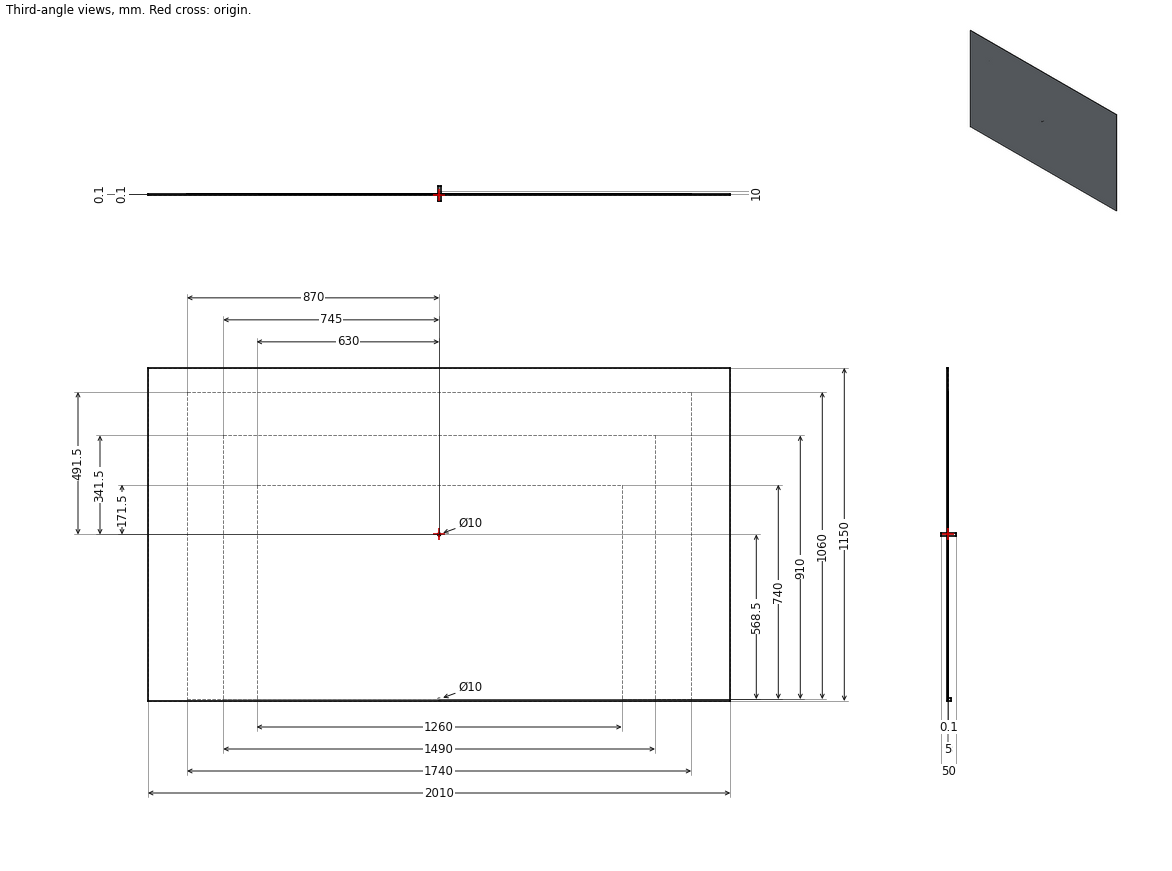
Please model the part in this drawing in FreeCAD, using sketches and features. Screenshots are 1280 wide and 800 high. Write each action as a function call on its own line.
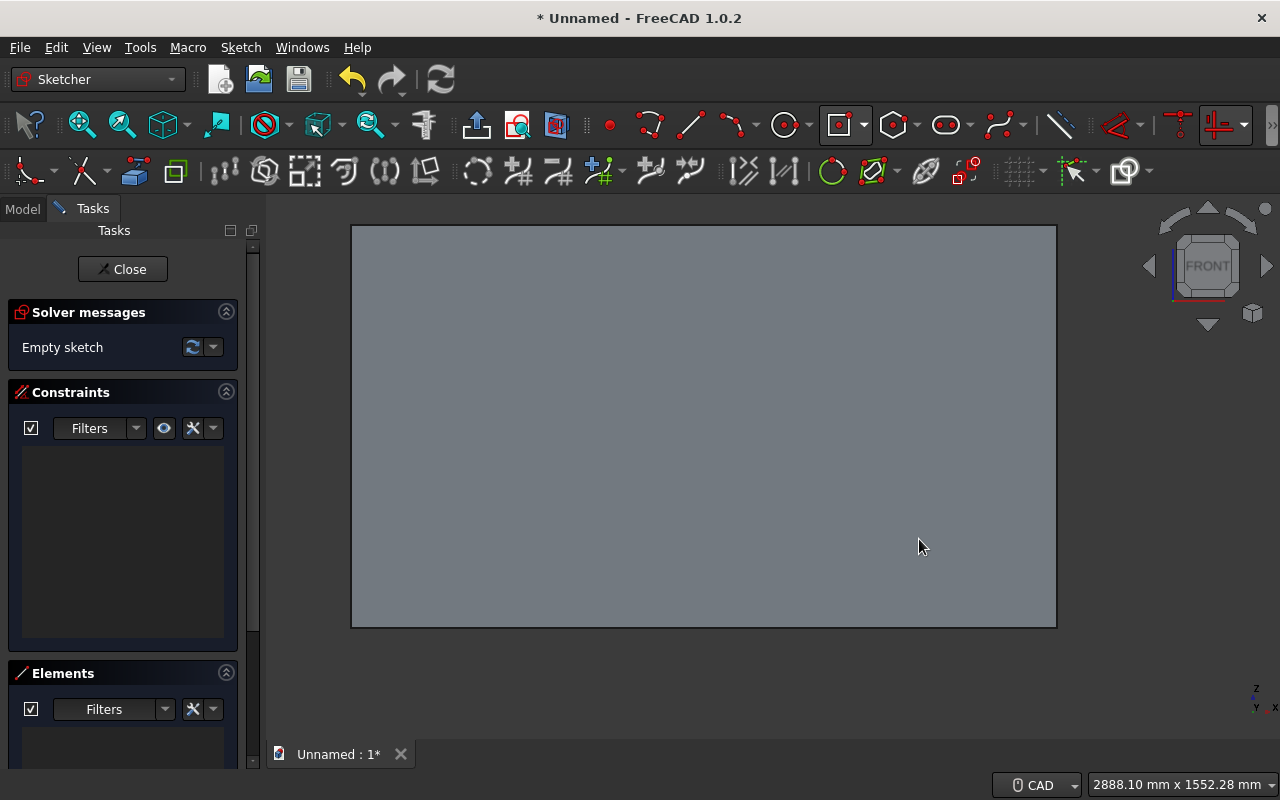
click(866, 126)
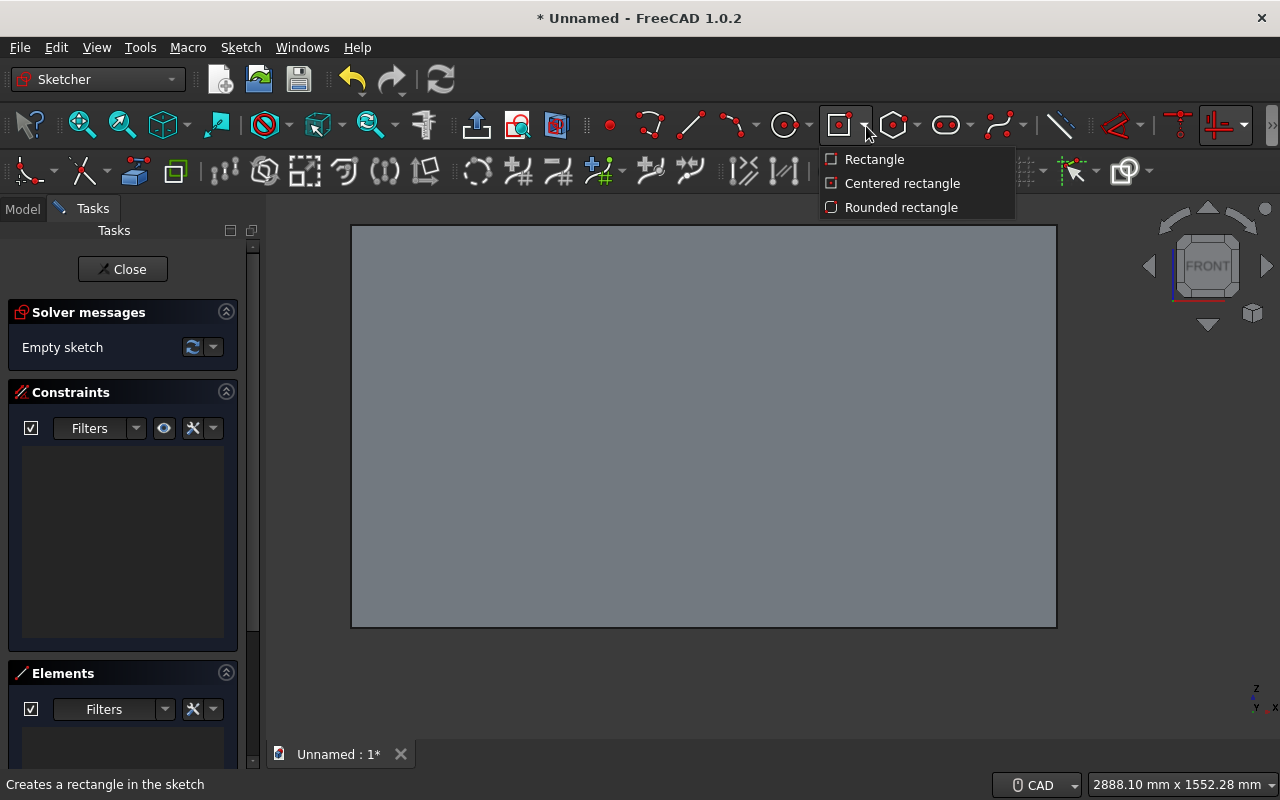
click(918, 159)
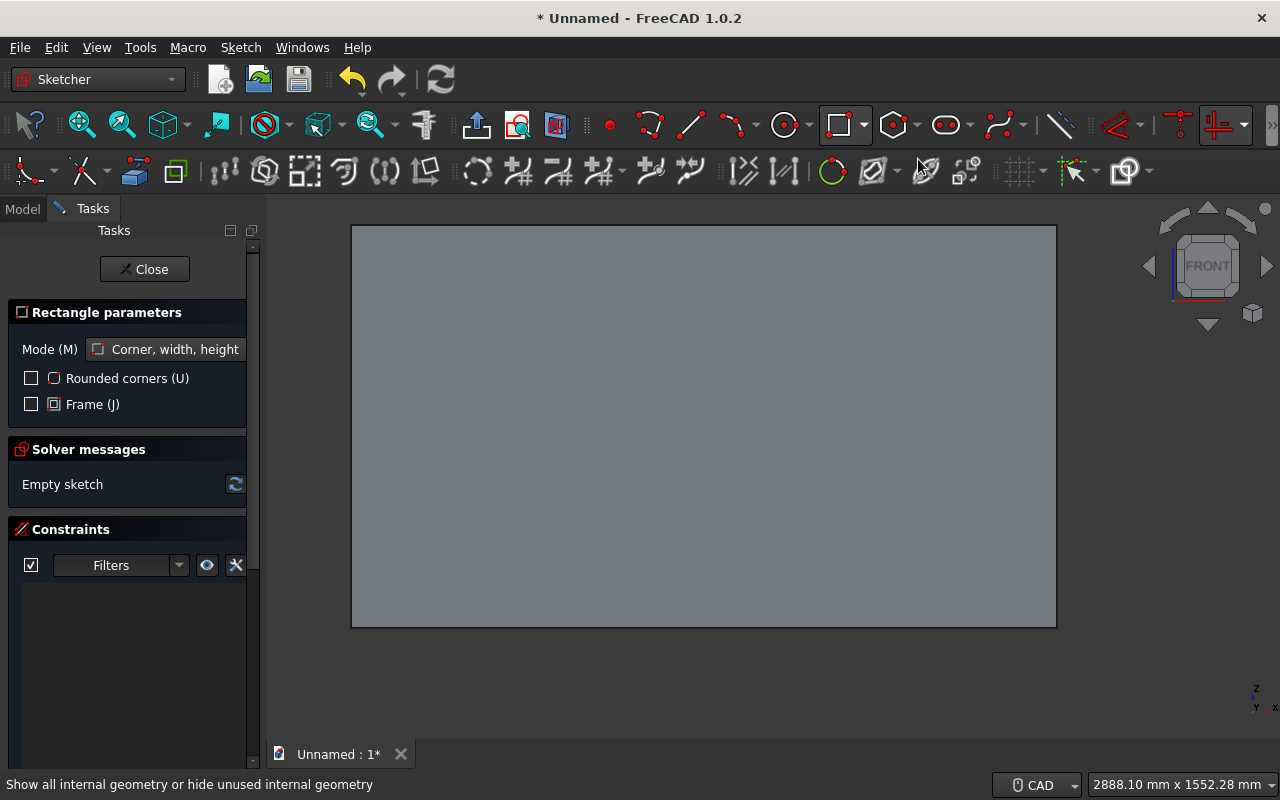
click(442, 307)
move(966, 626)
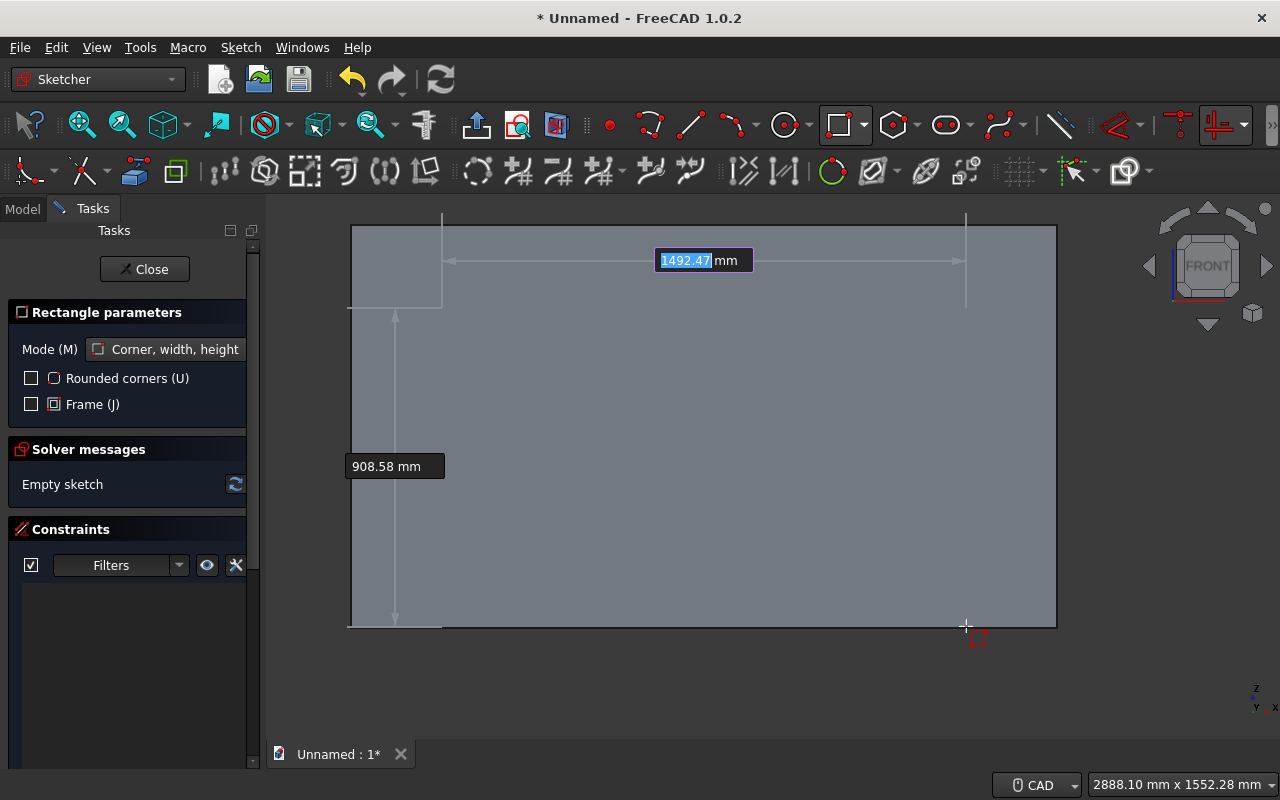
text(1490)
key(Tab)
text(910)
key(Return)
key(Escape)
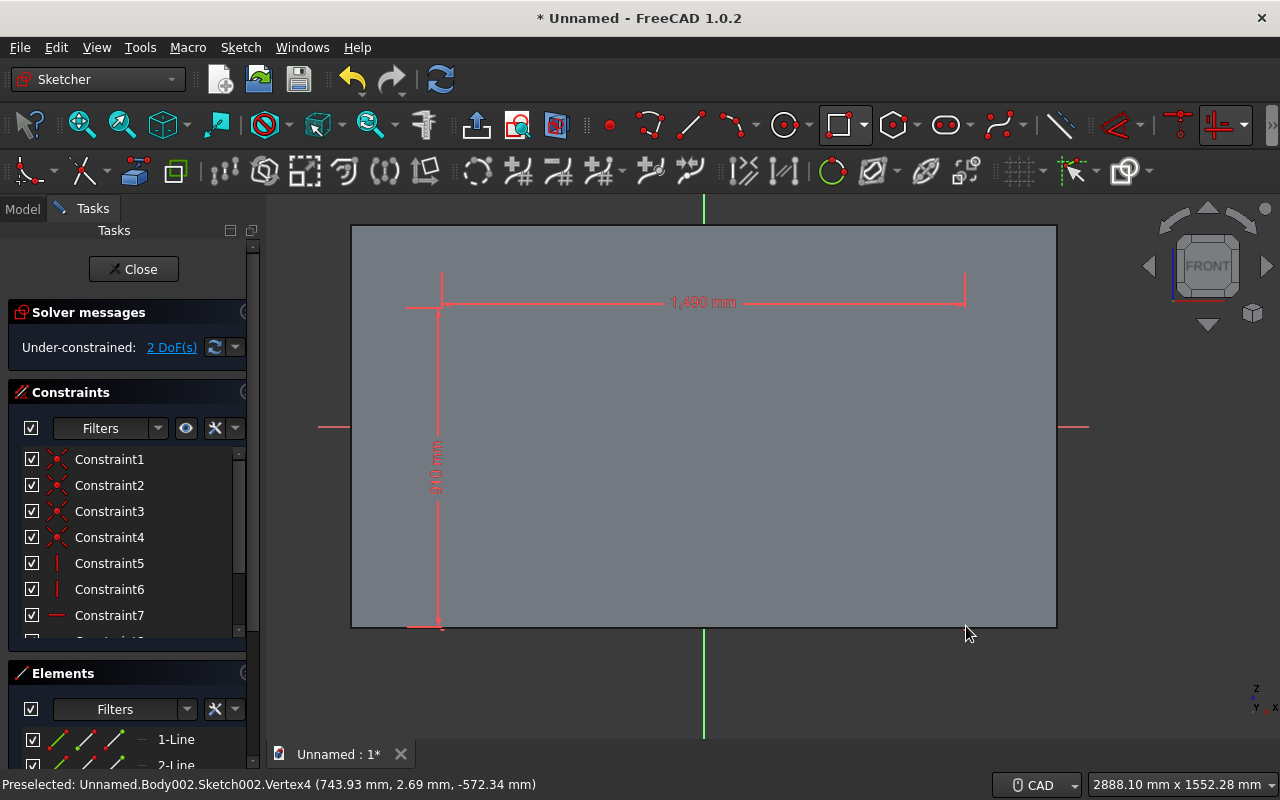
click(1116, 126)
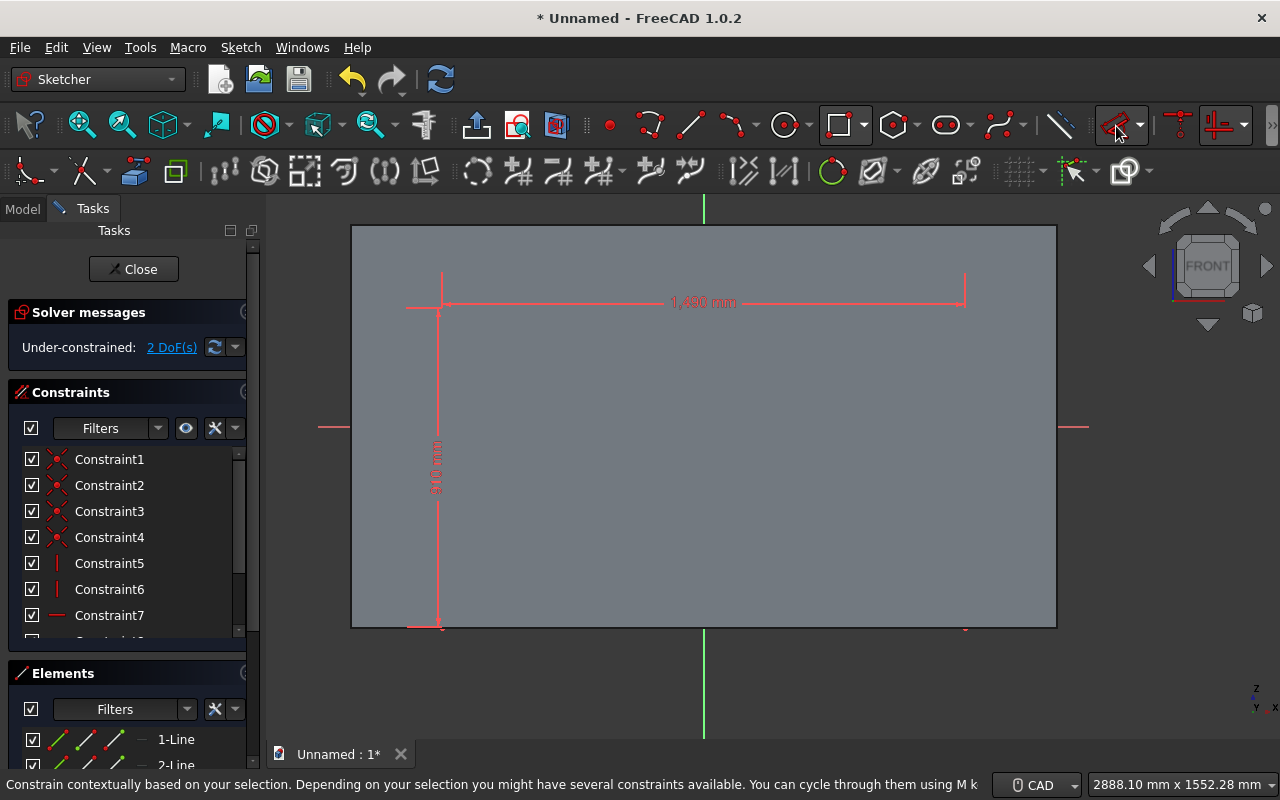
click(442, 308)
click(573, 274)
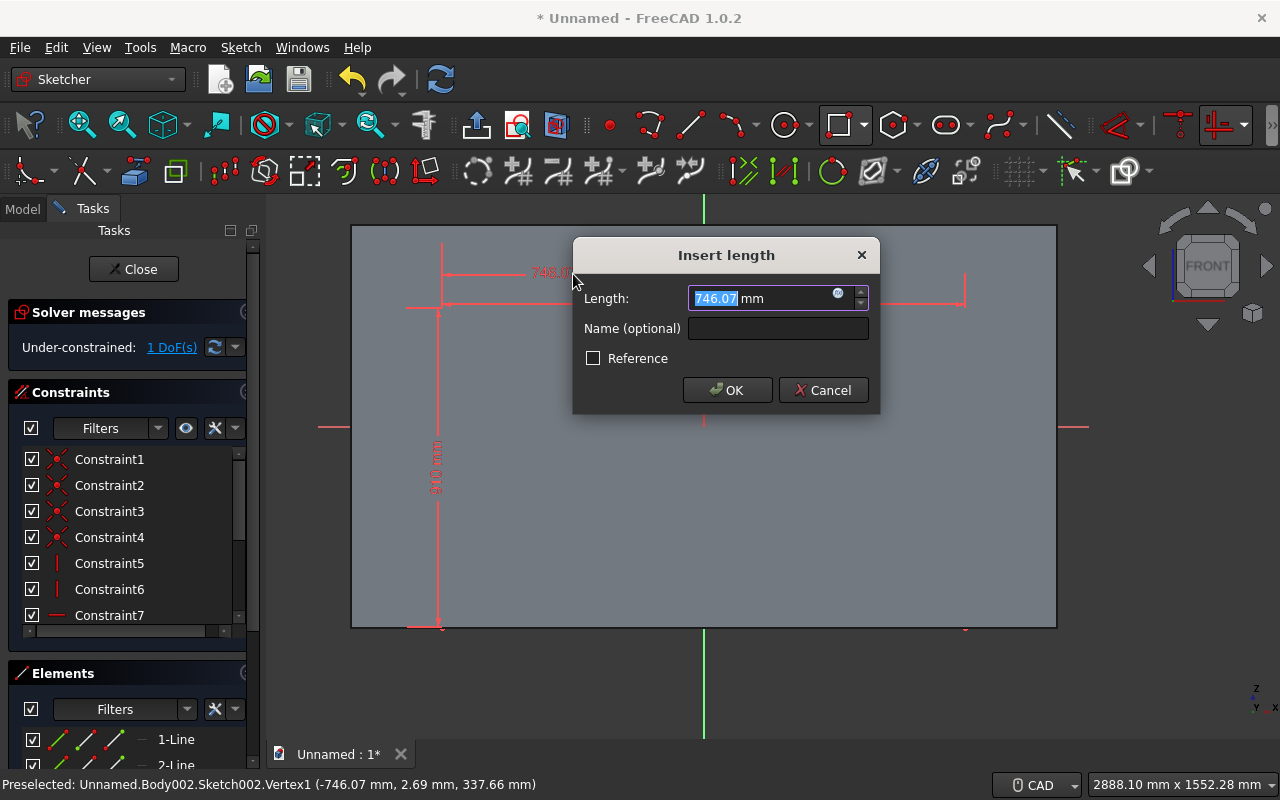
text(745)
key(Return)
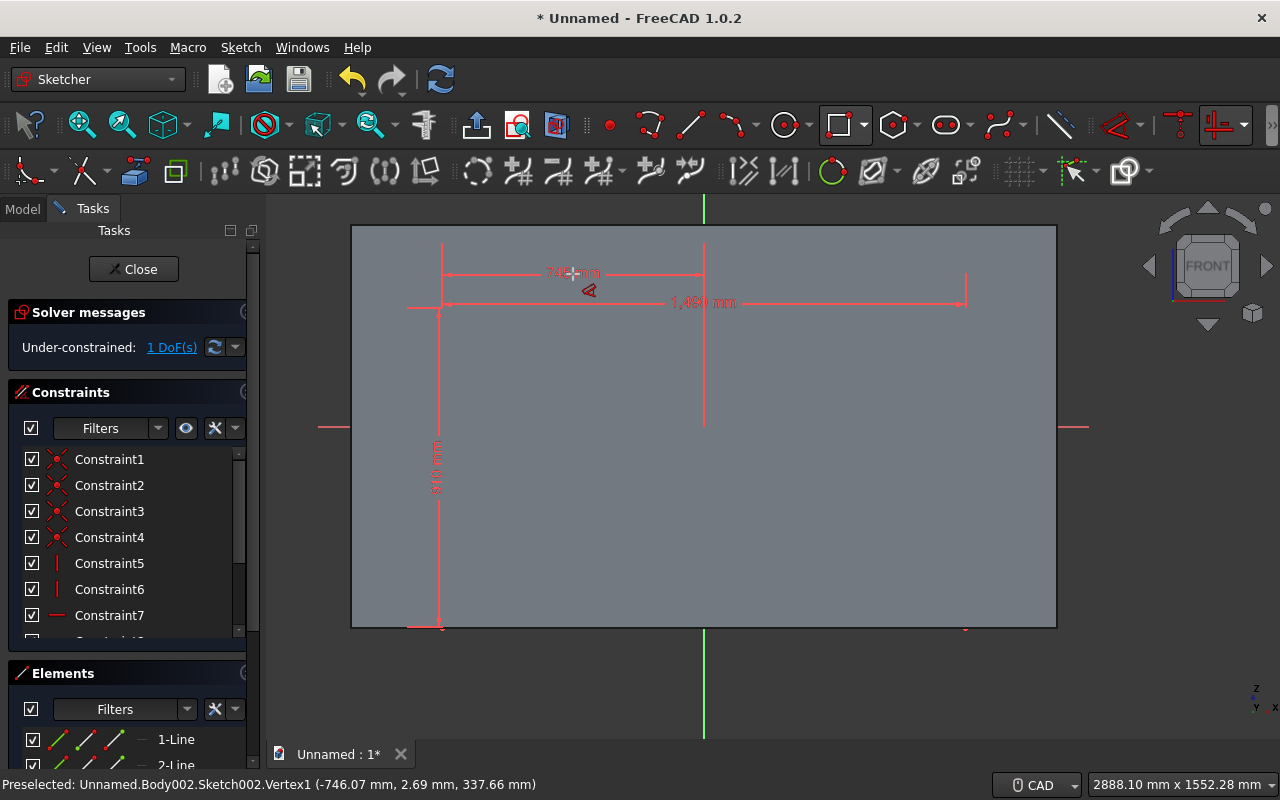
click(442, 308)
click(408, 367)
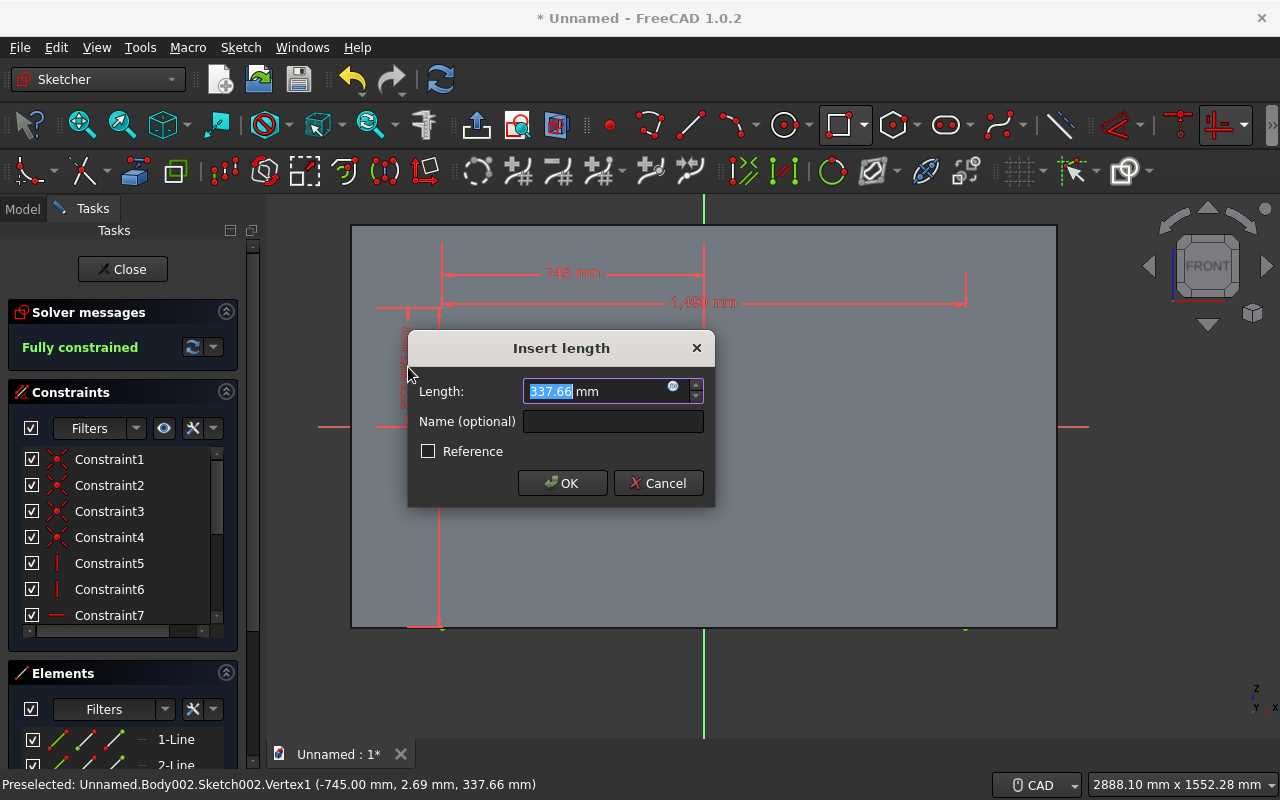
text(341.5)
key(Return)
key(Escape)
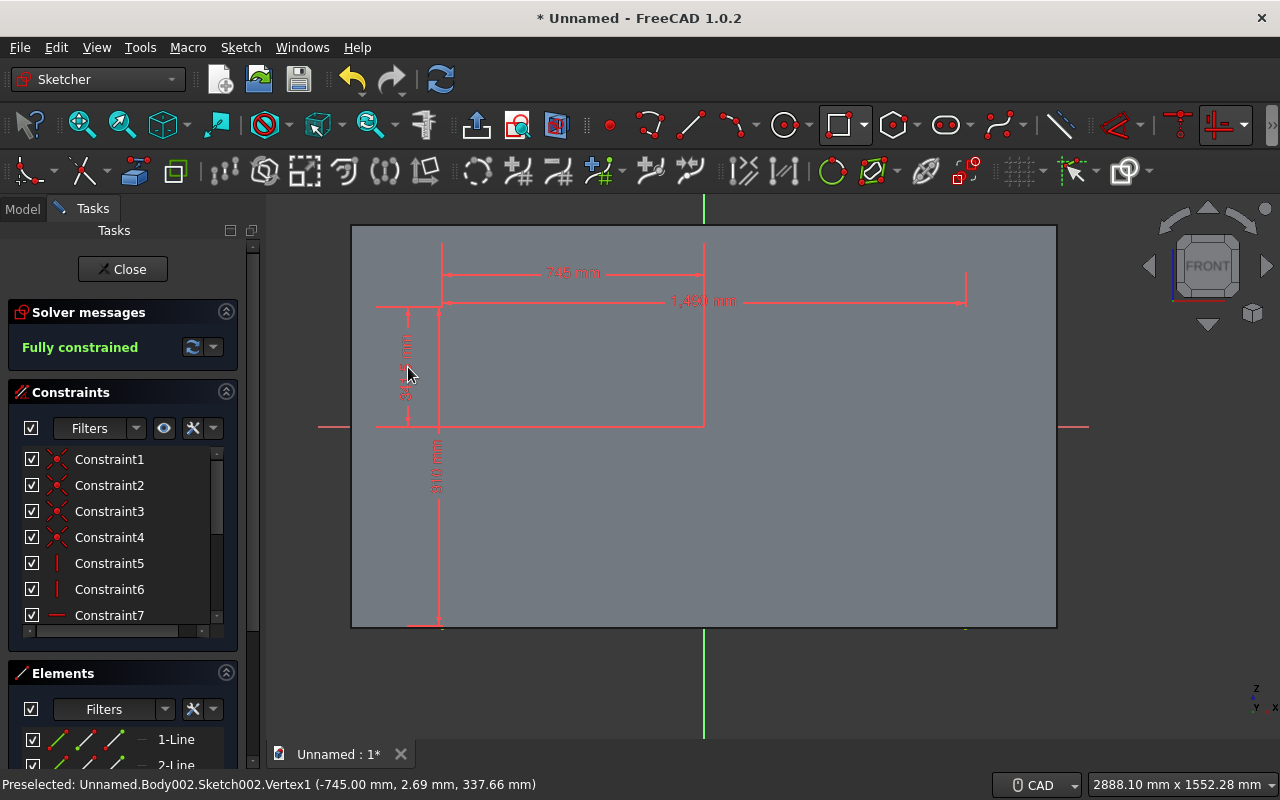
click(123, 269)